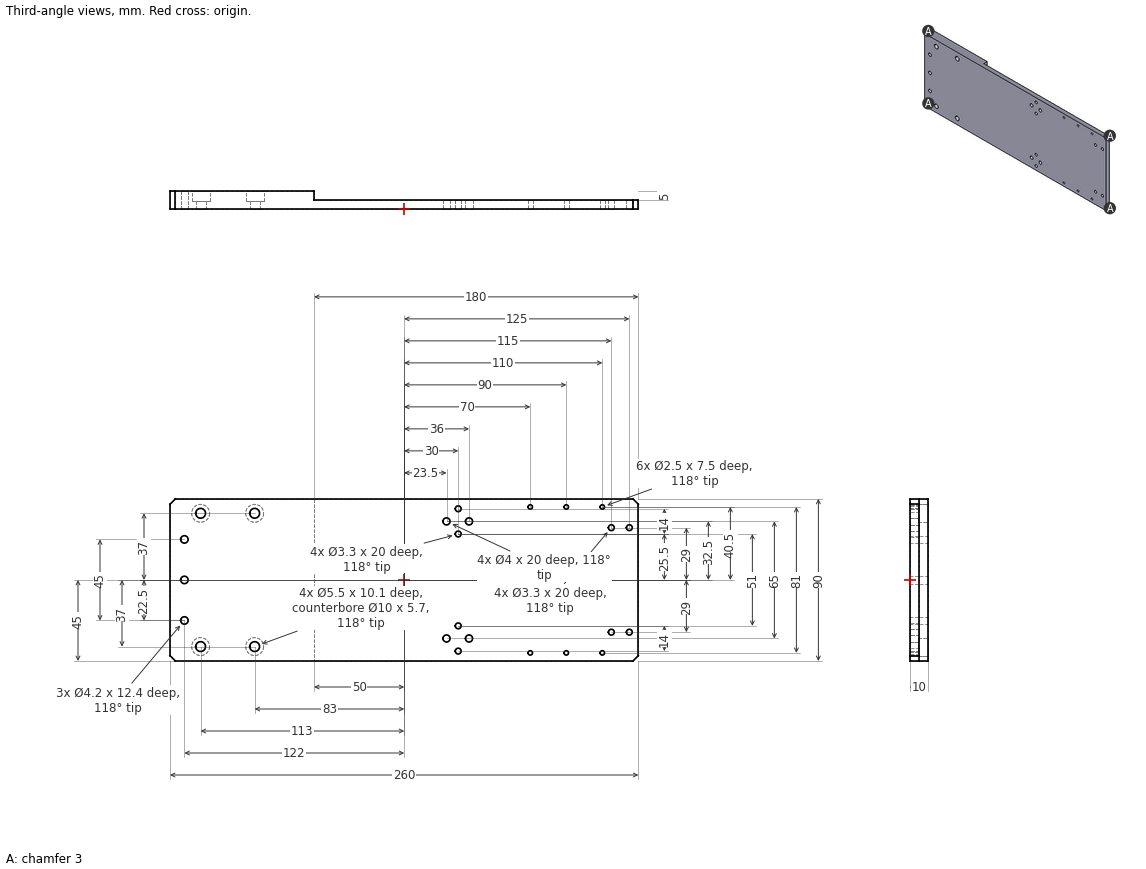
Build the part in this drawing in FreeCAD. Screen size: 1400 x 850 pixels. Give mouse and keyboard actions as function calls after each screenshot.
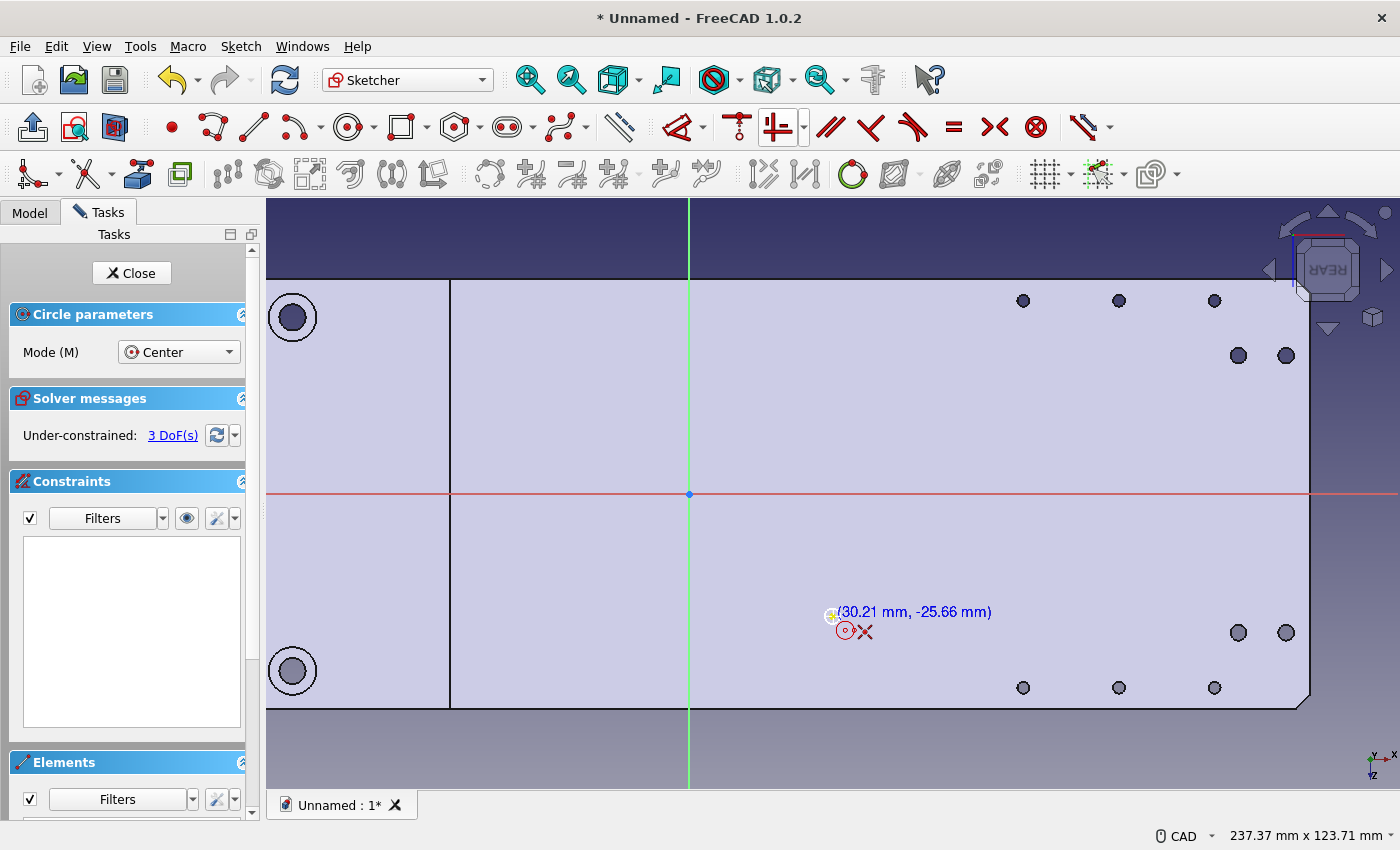
scroll(832, 683, up, 6)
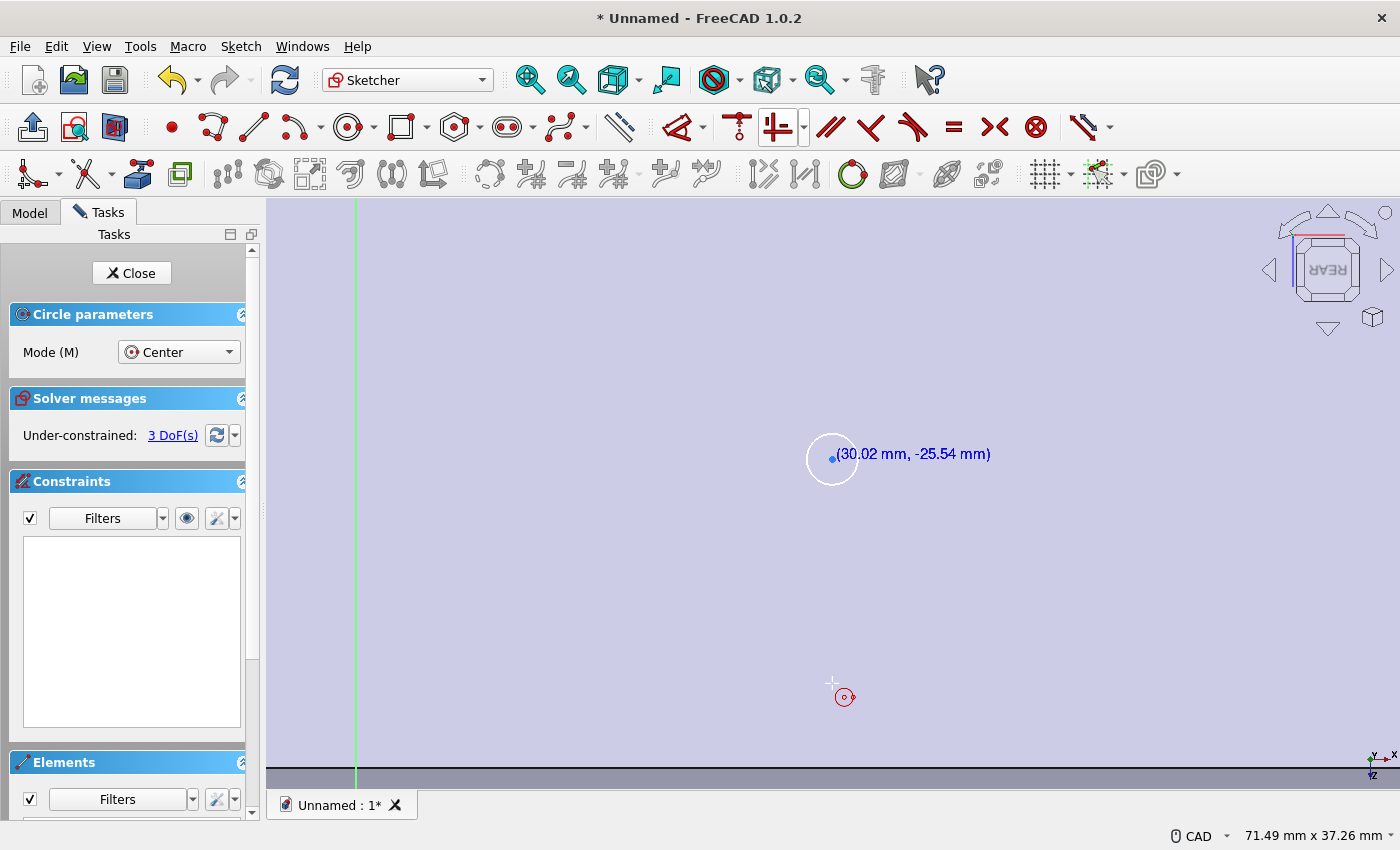
click(832, 681)
click(851, 662)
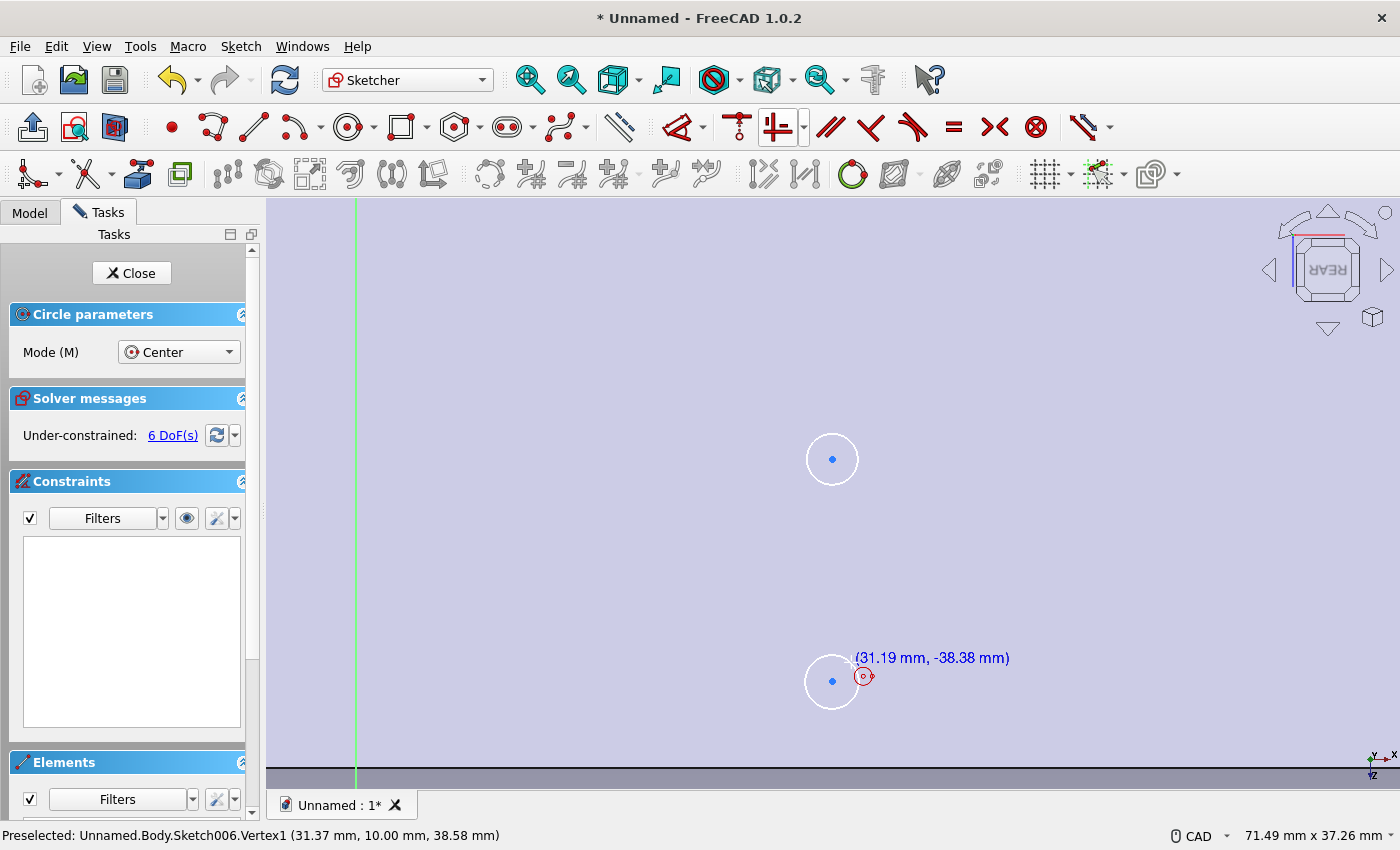
scroll(832, 683, down, 6)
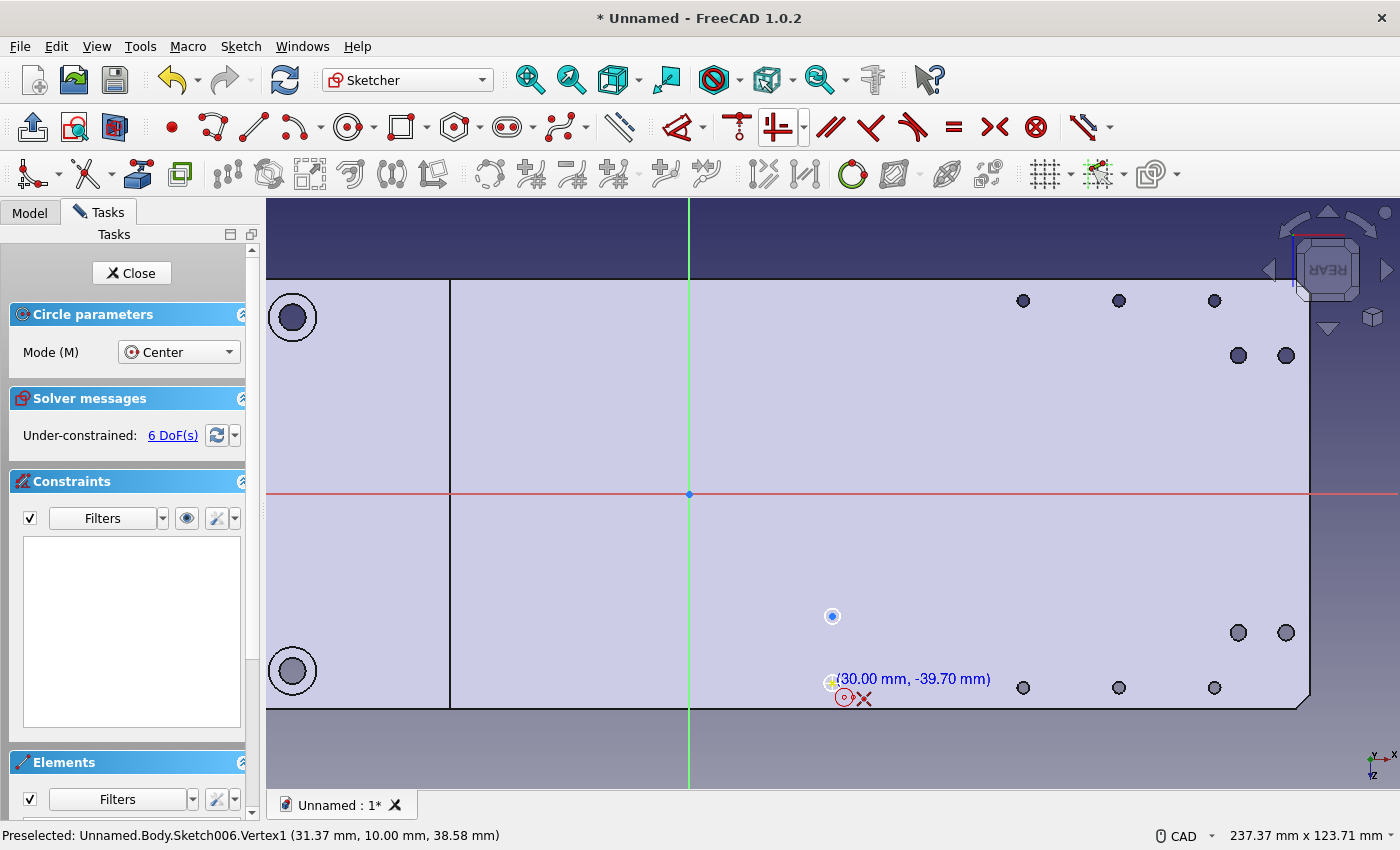
scroll(832, 372, up, 6)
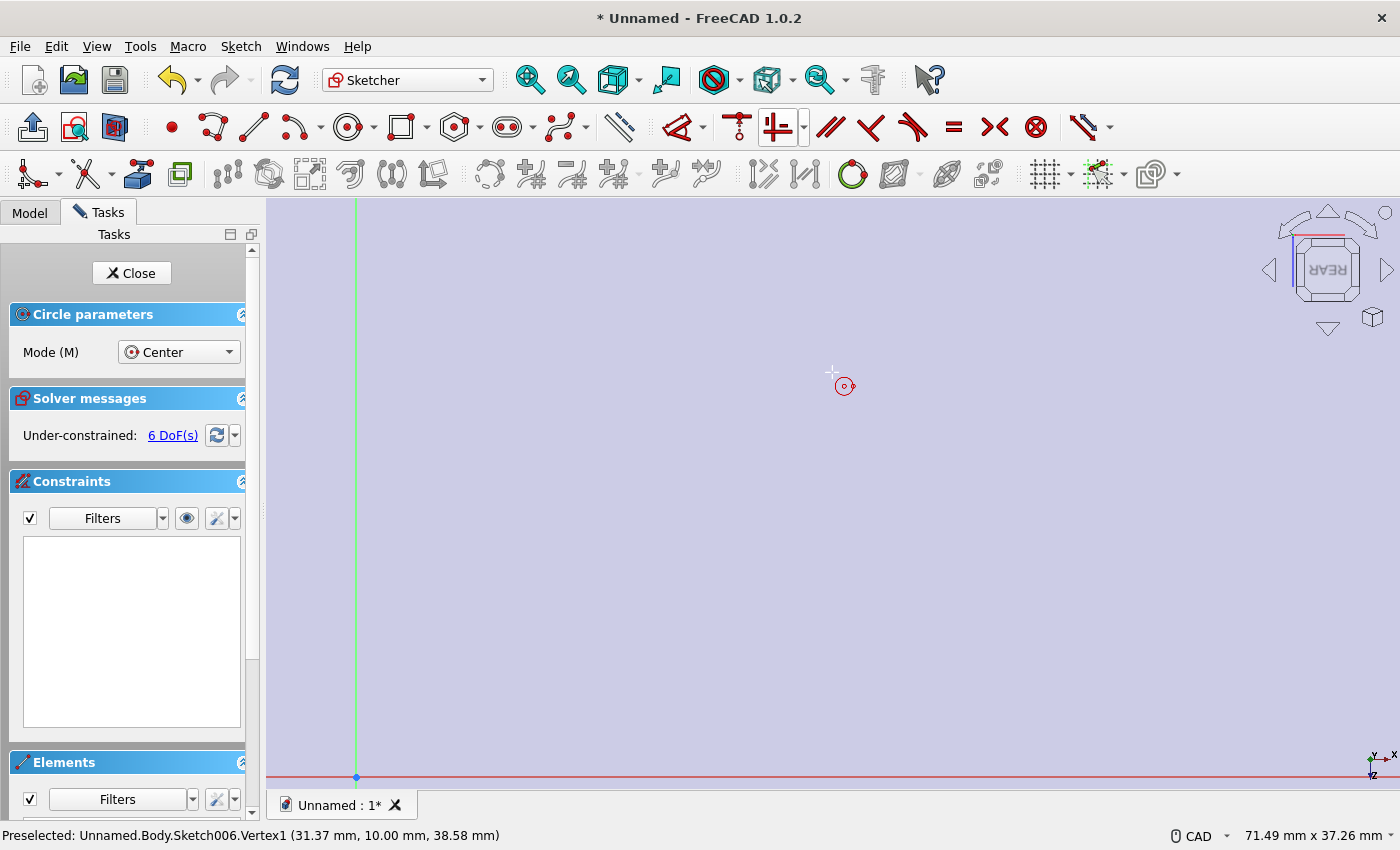
click(832, 373)
click(851, 354)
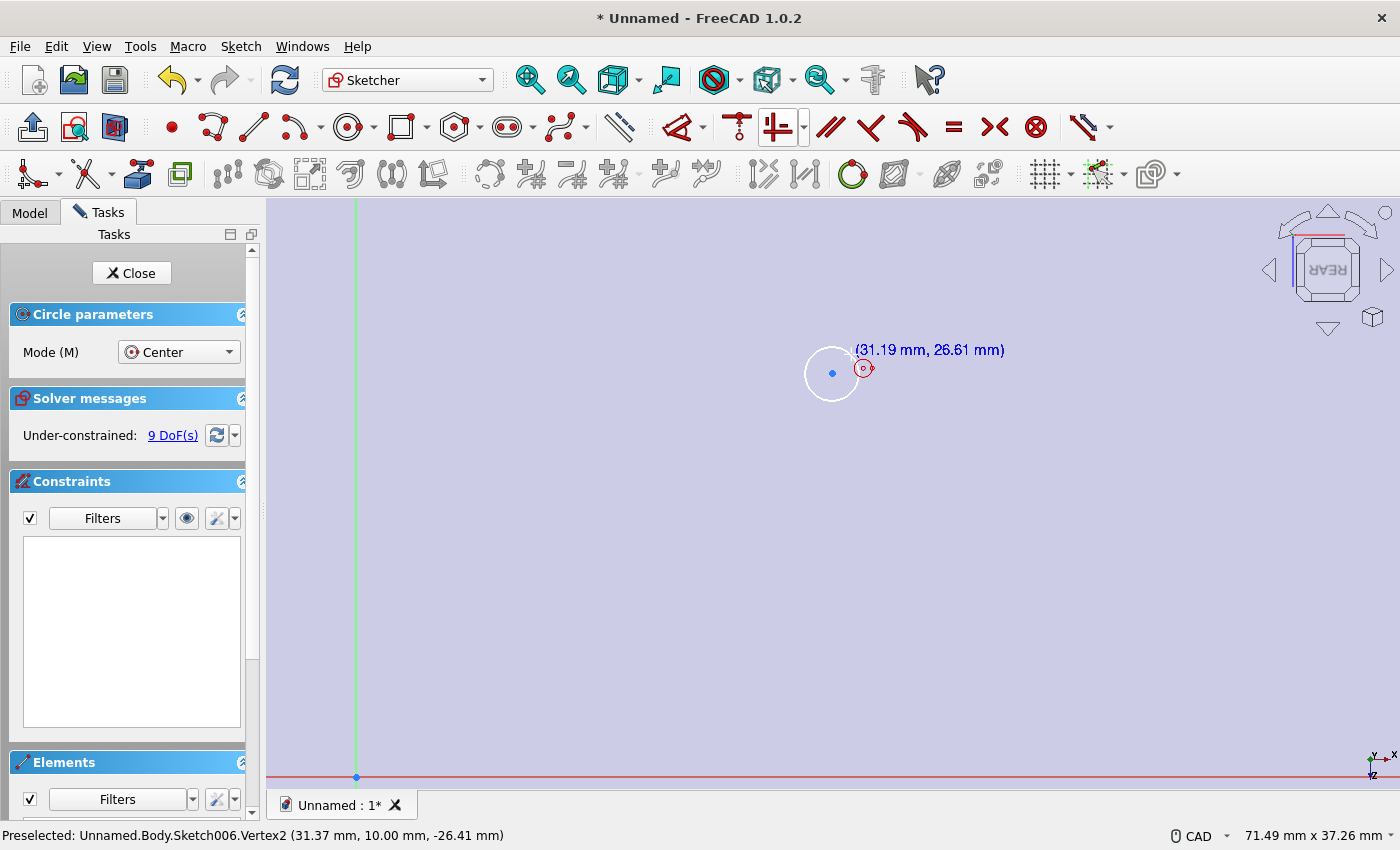
scroll(832, 371, down, 6)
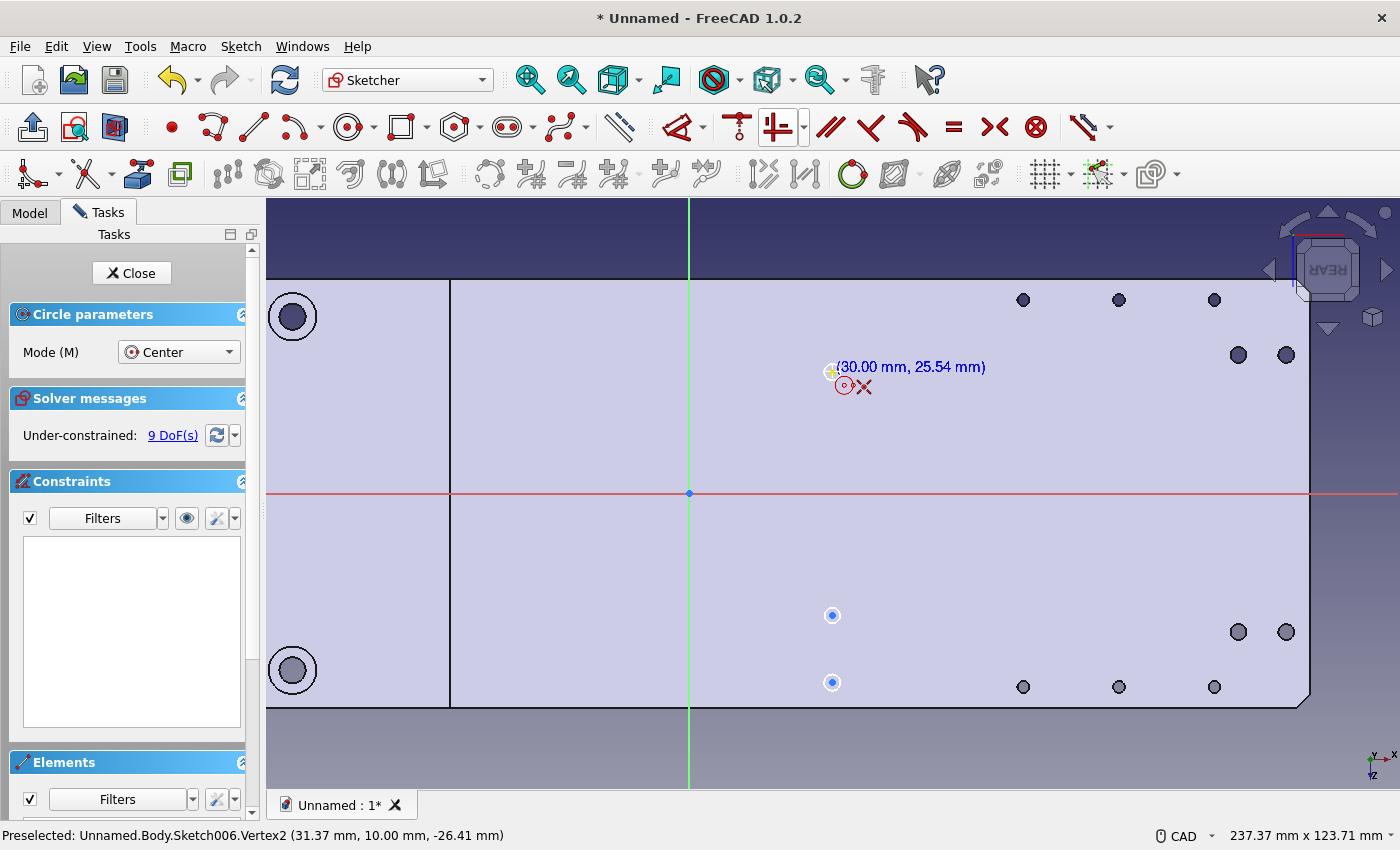
scroll(832, 305, up, 6)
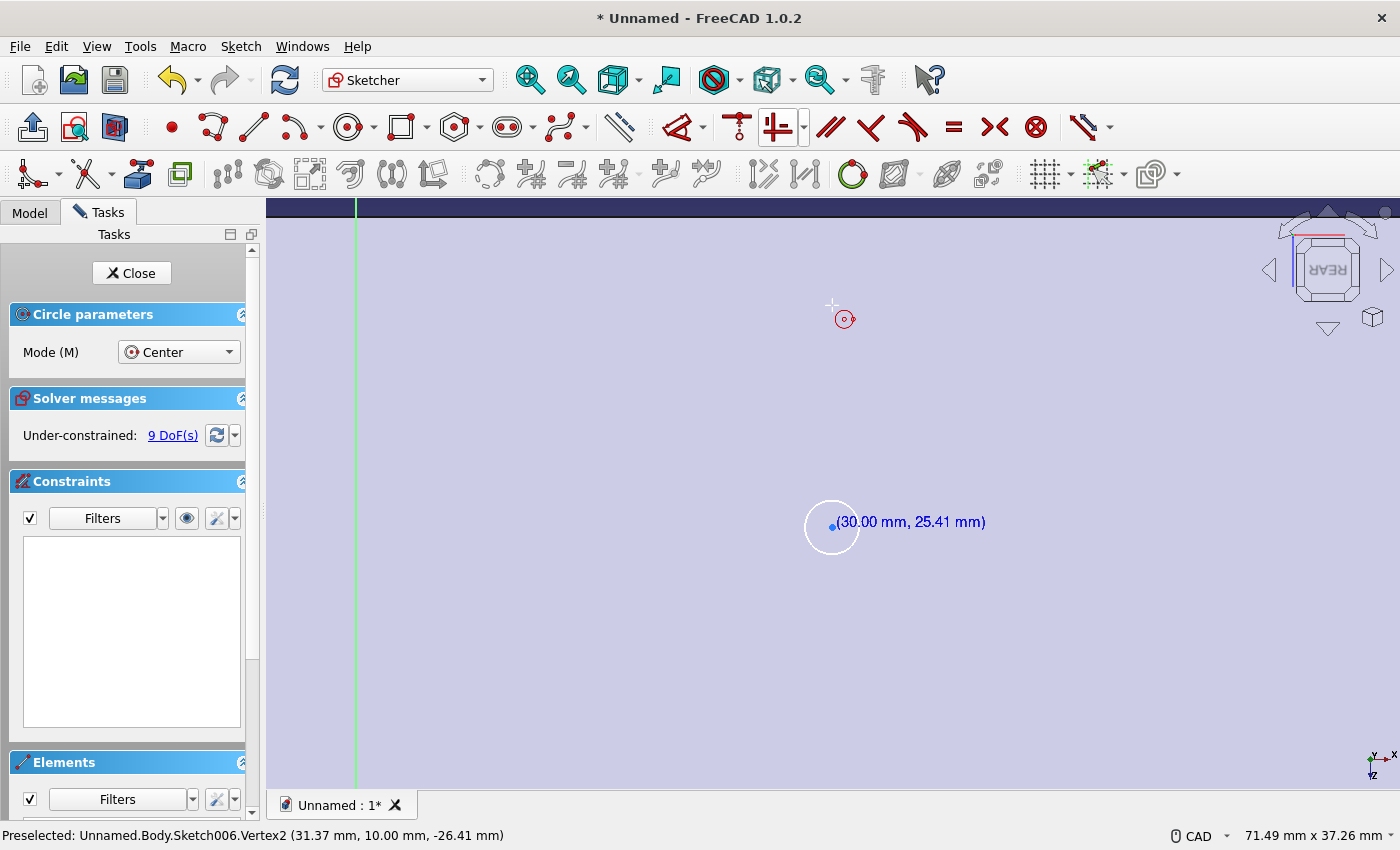
click(832, 304)
click(851, 285)
key(Escape)